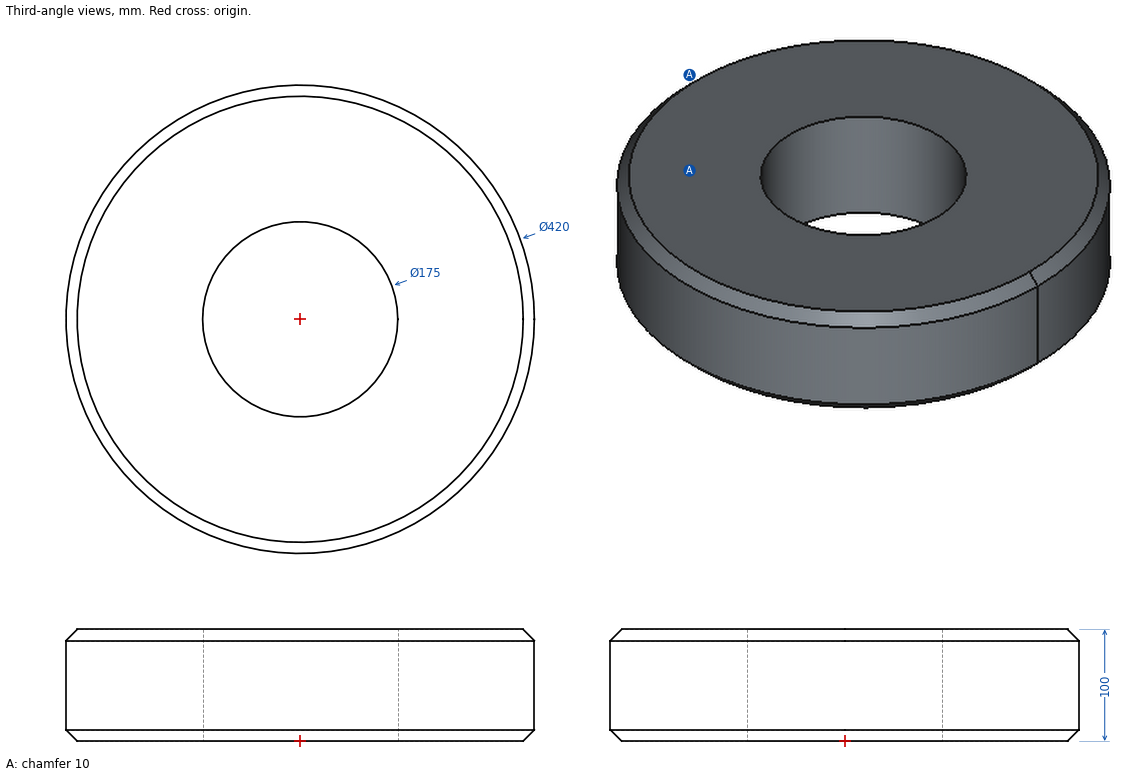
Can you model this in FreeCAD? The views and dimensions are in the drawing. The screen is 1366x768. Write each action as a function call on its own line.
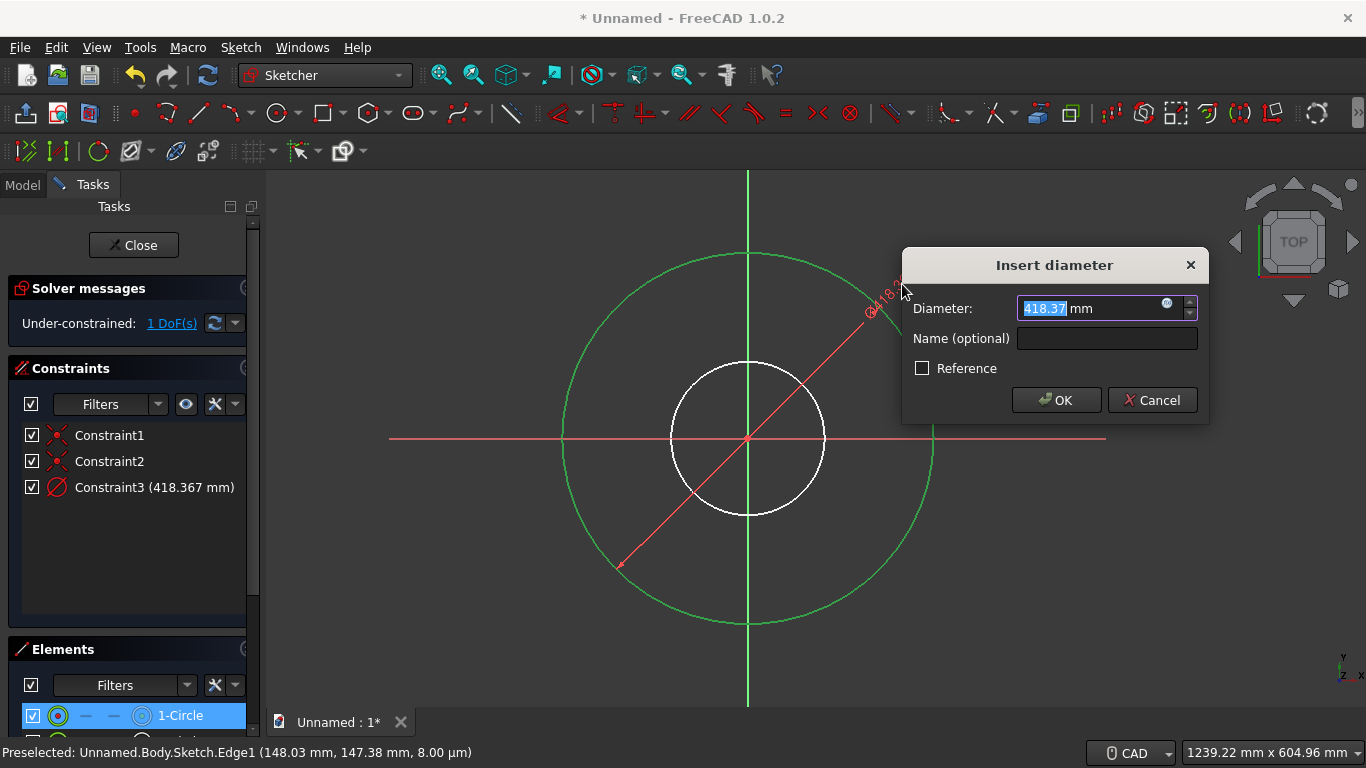
text(420)
key(Return)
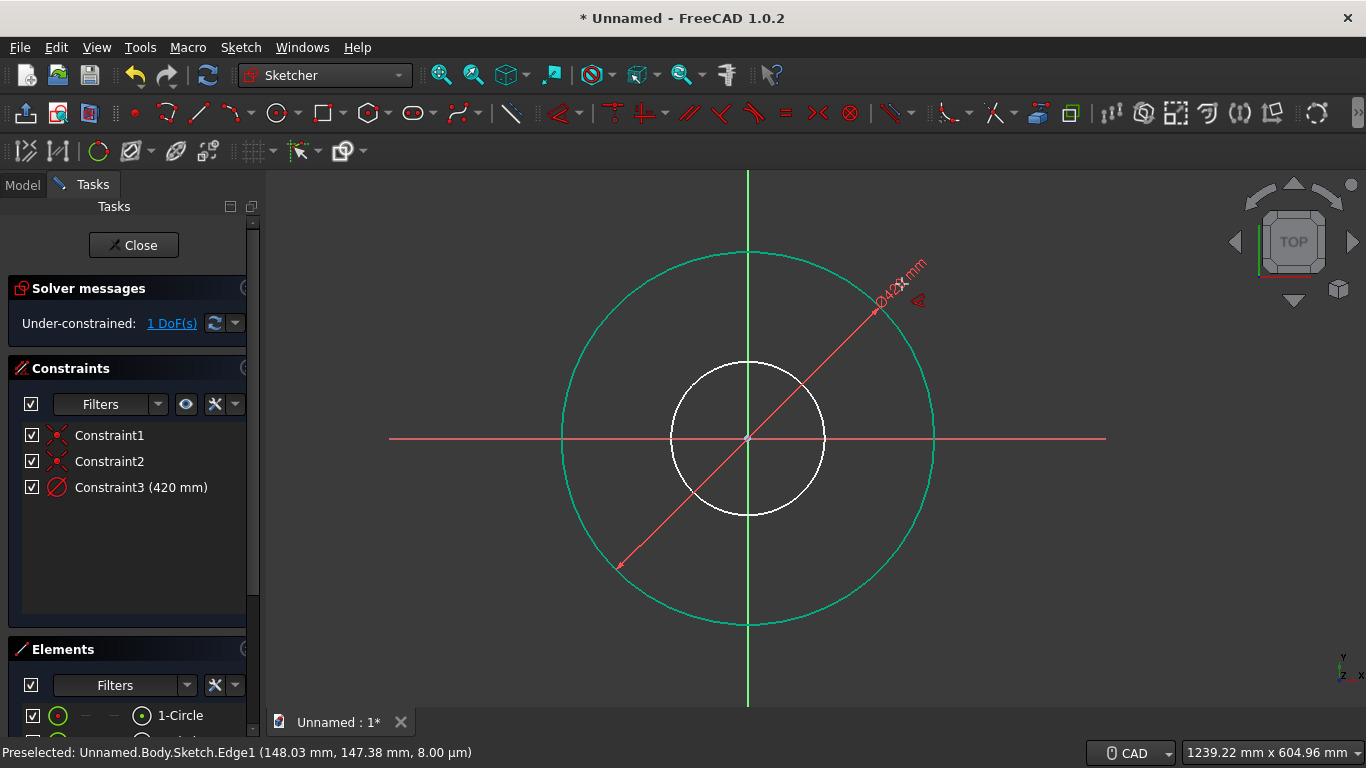
click(802, 384)
click(825, 361)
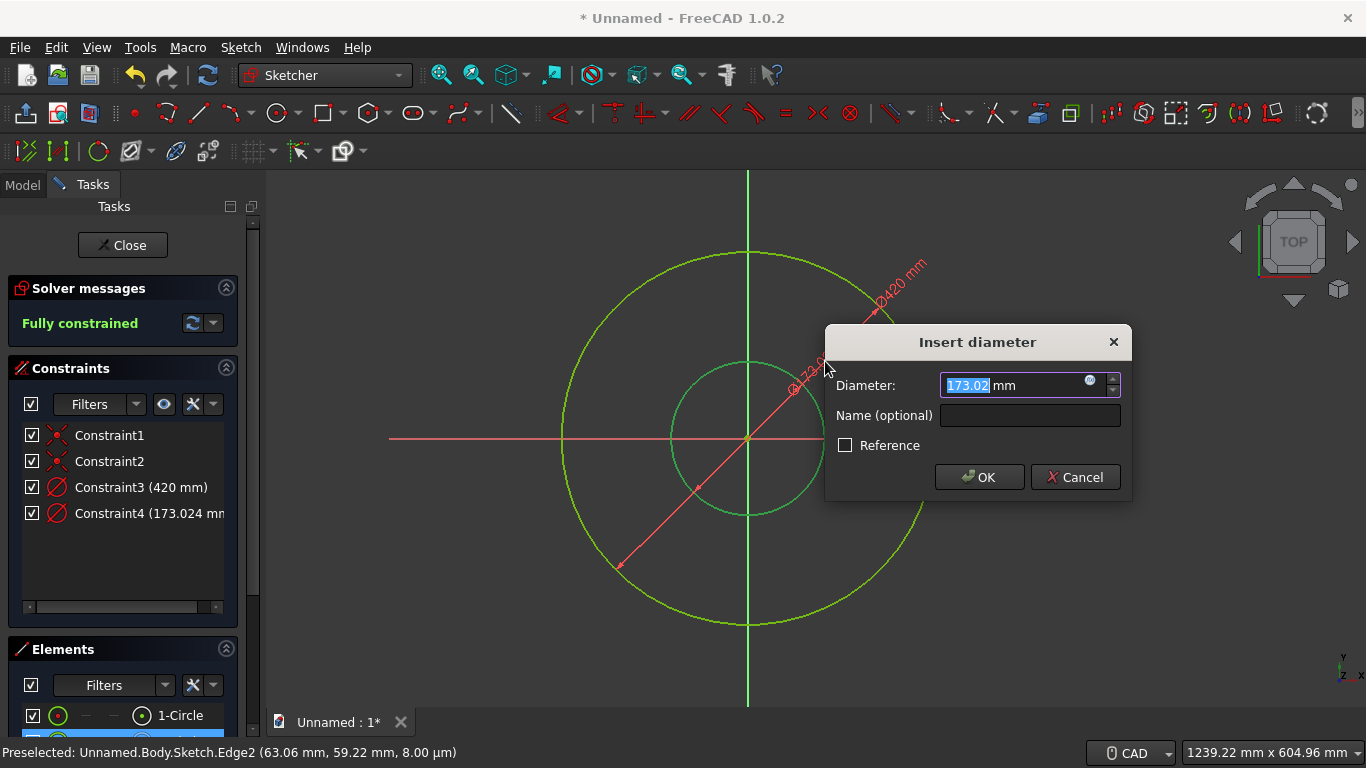
text(175)
key(Return)
key(Escape)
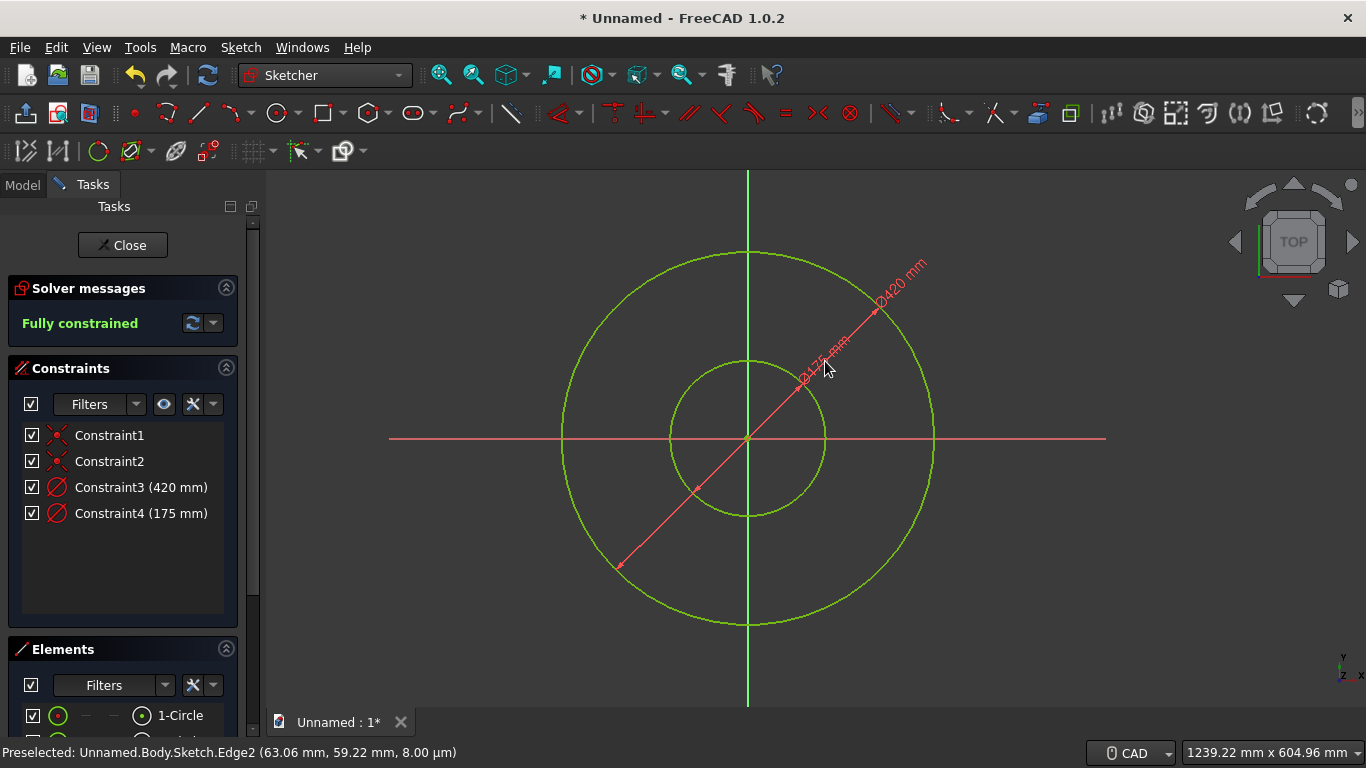
click(123, 245)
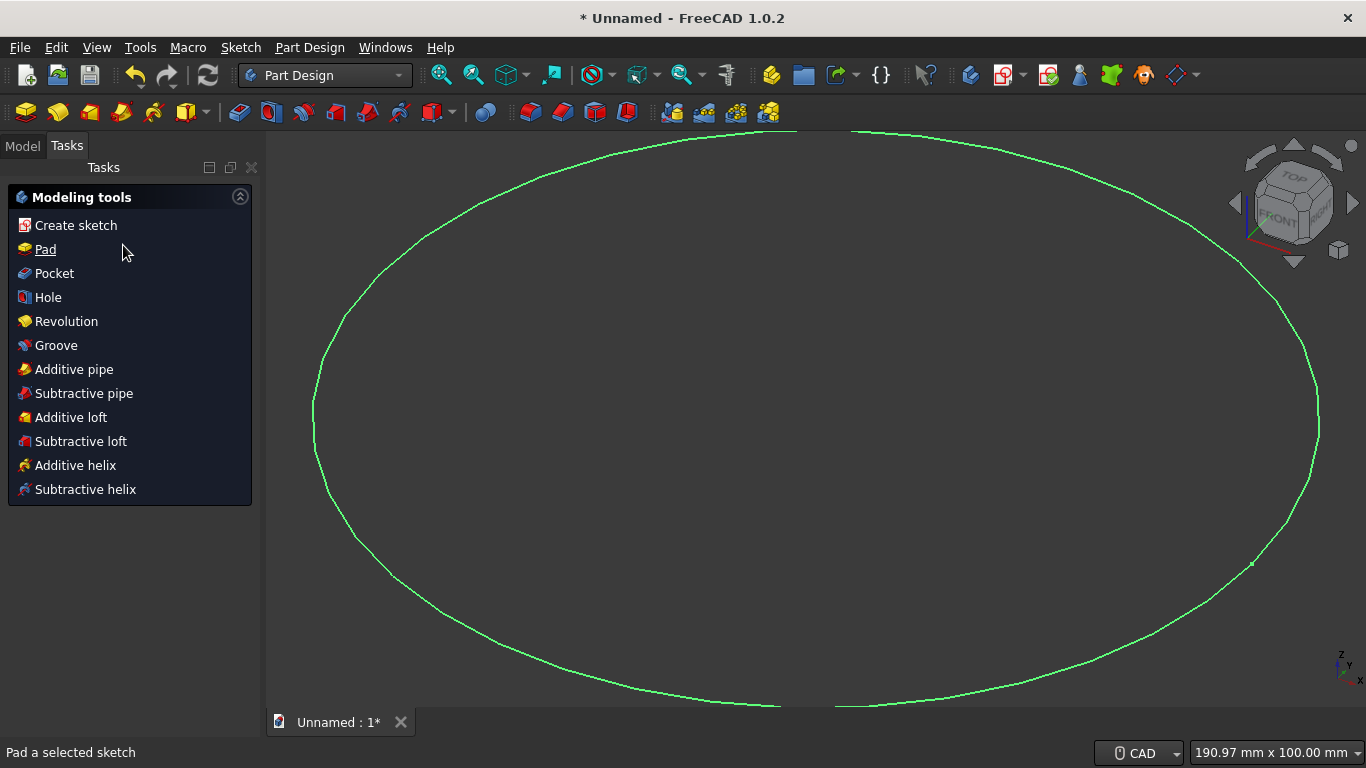
click(26, 112)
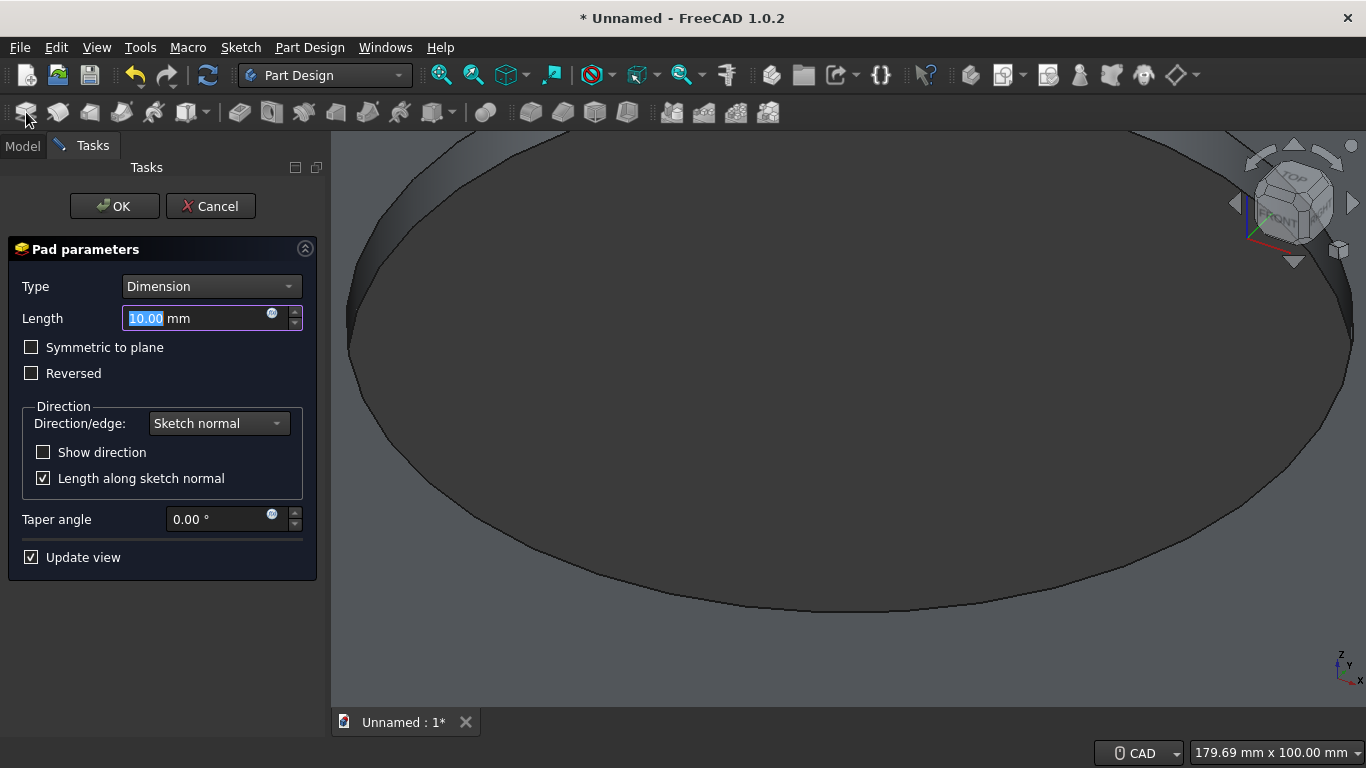
text(100)
key(Tab)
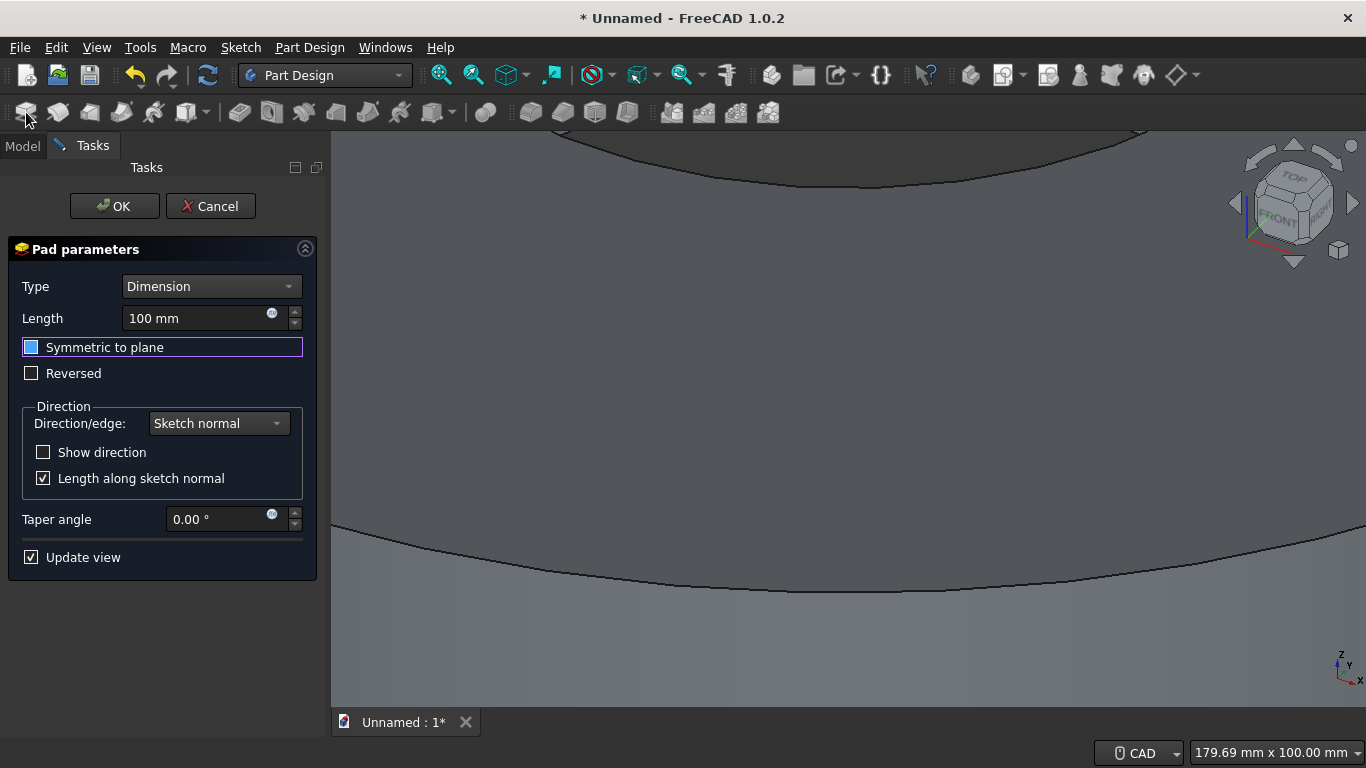
click(115, 206)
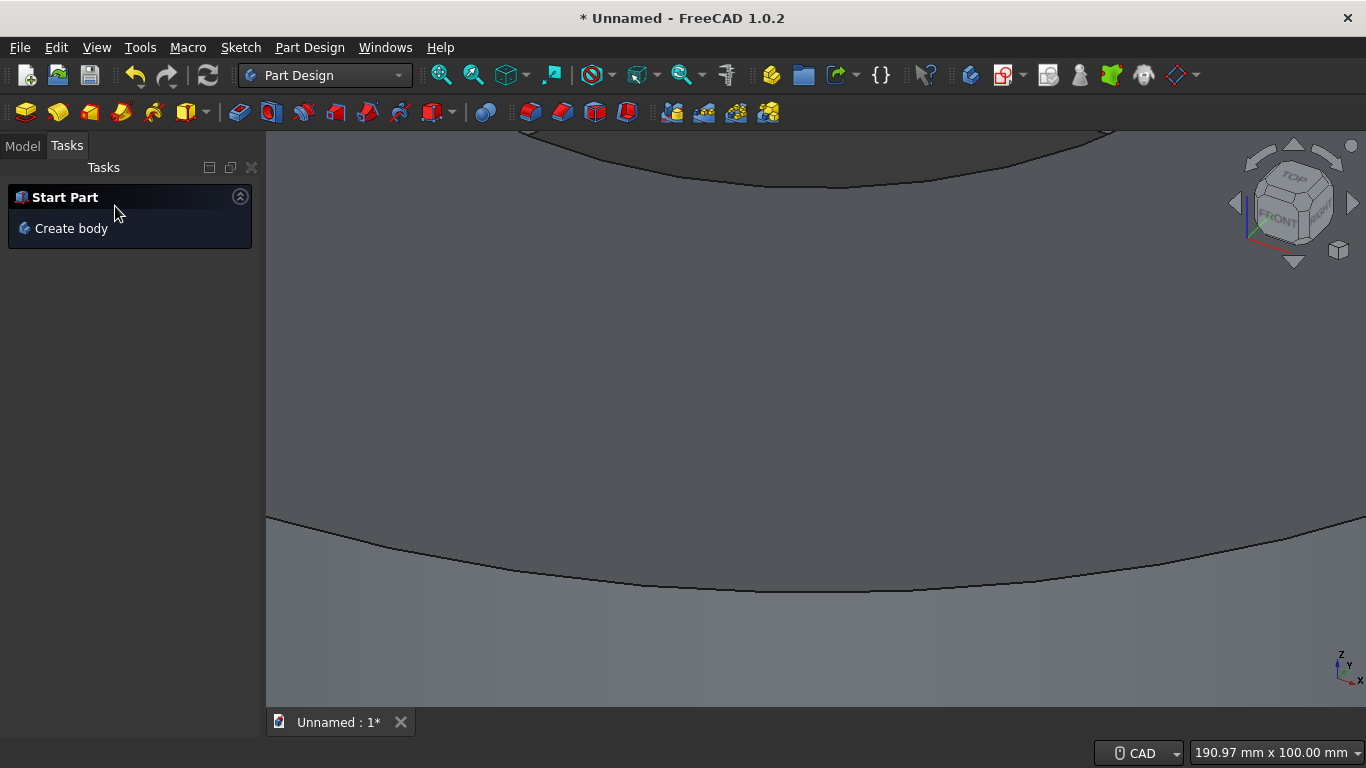
click(442, 76)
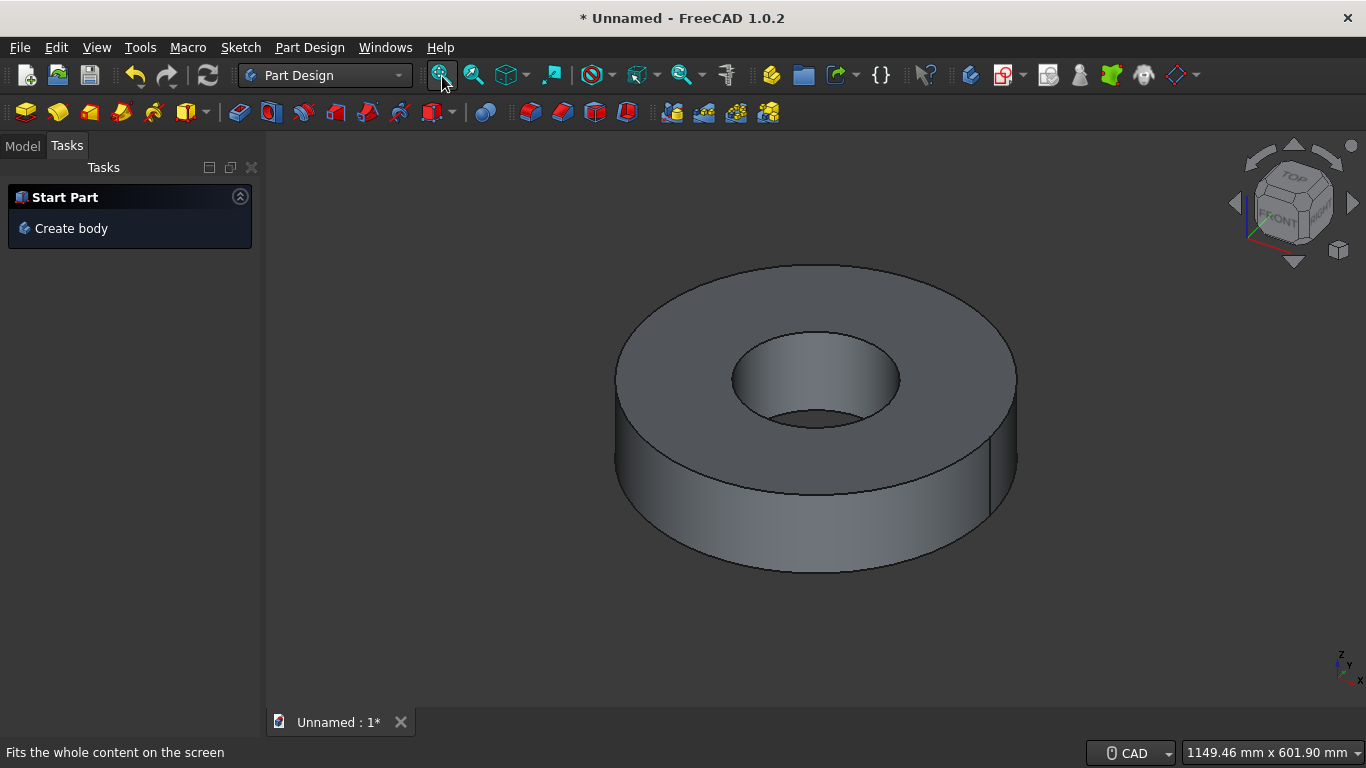
click(616, 391)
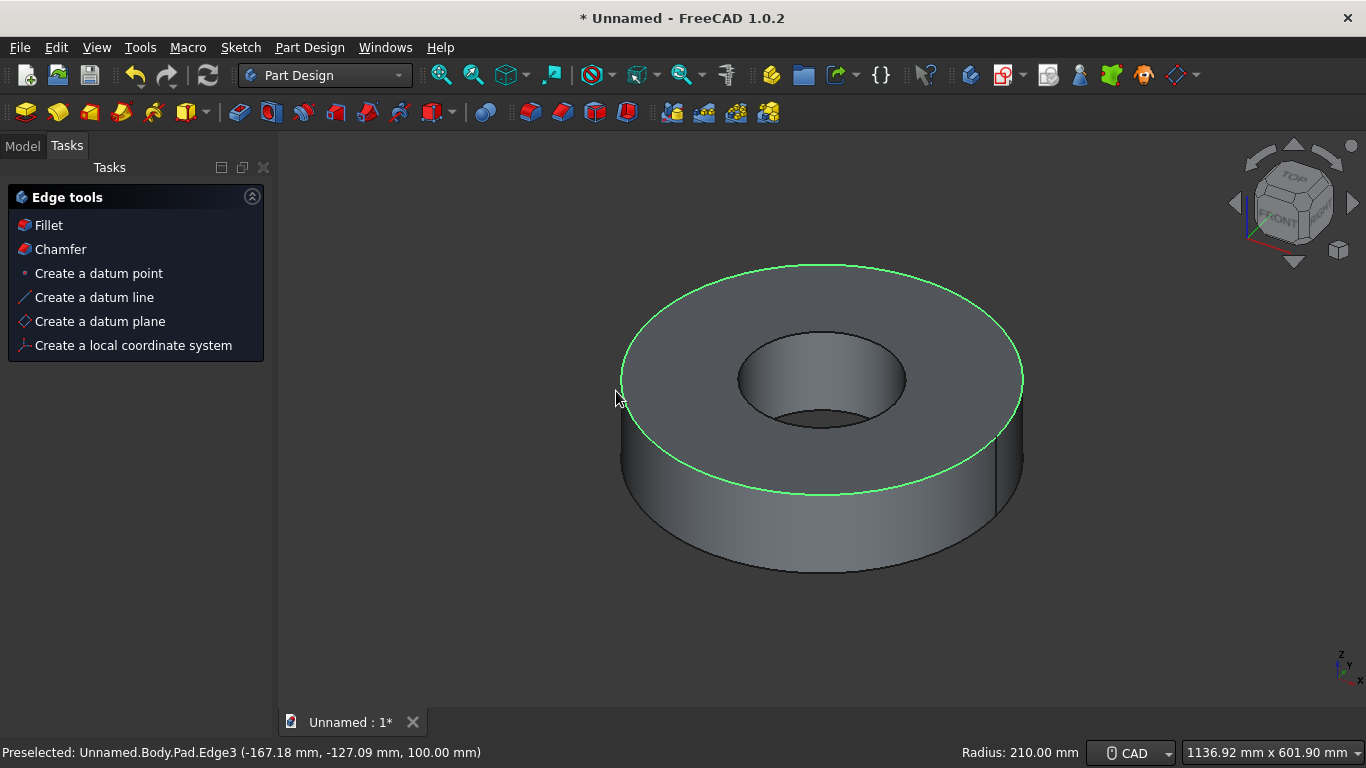
key(0)